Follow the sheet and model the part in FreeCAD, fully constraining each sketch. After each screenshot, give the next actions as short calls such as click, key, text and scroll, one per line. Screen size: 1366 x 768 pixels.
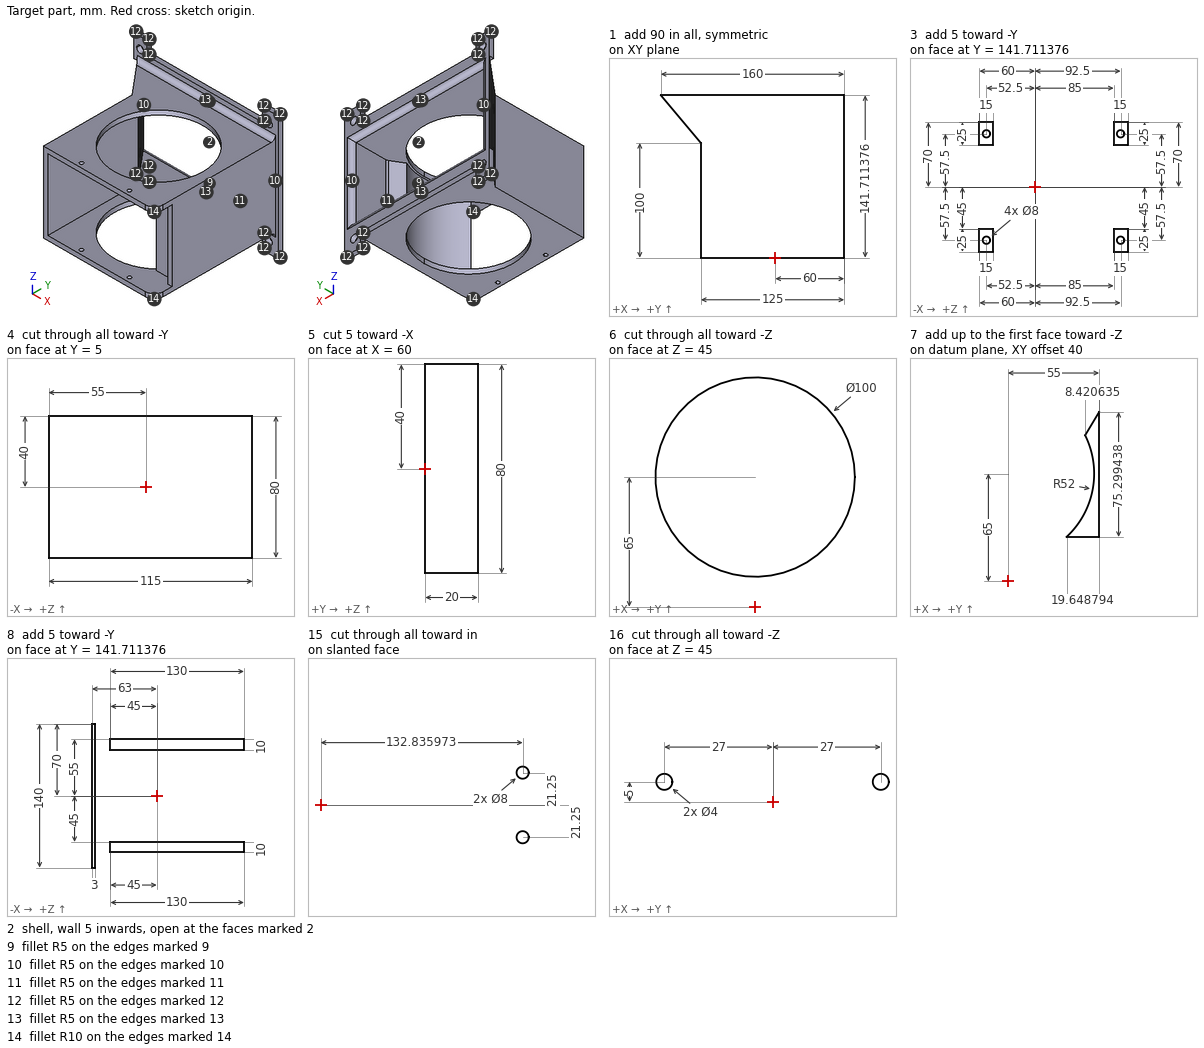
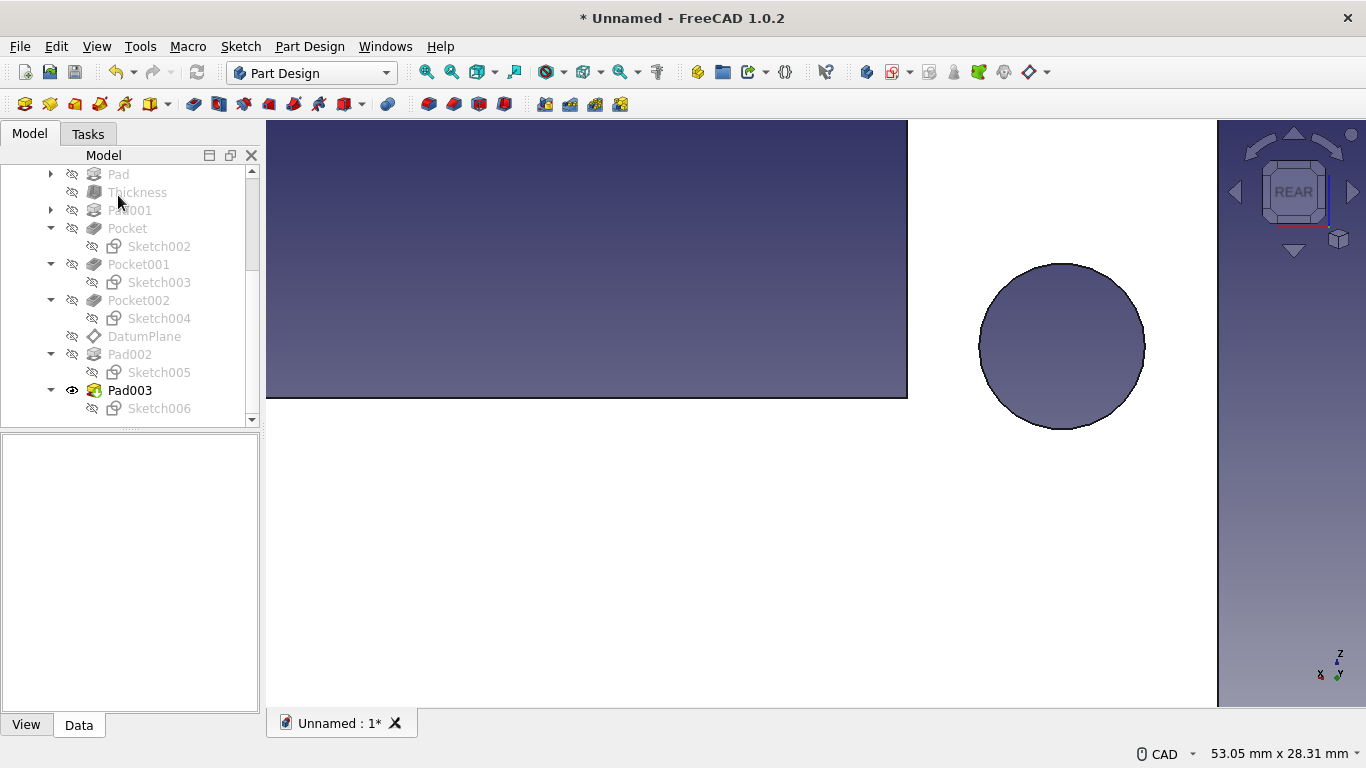
click(427, 72)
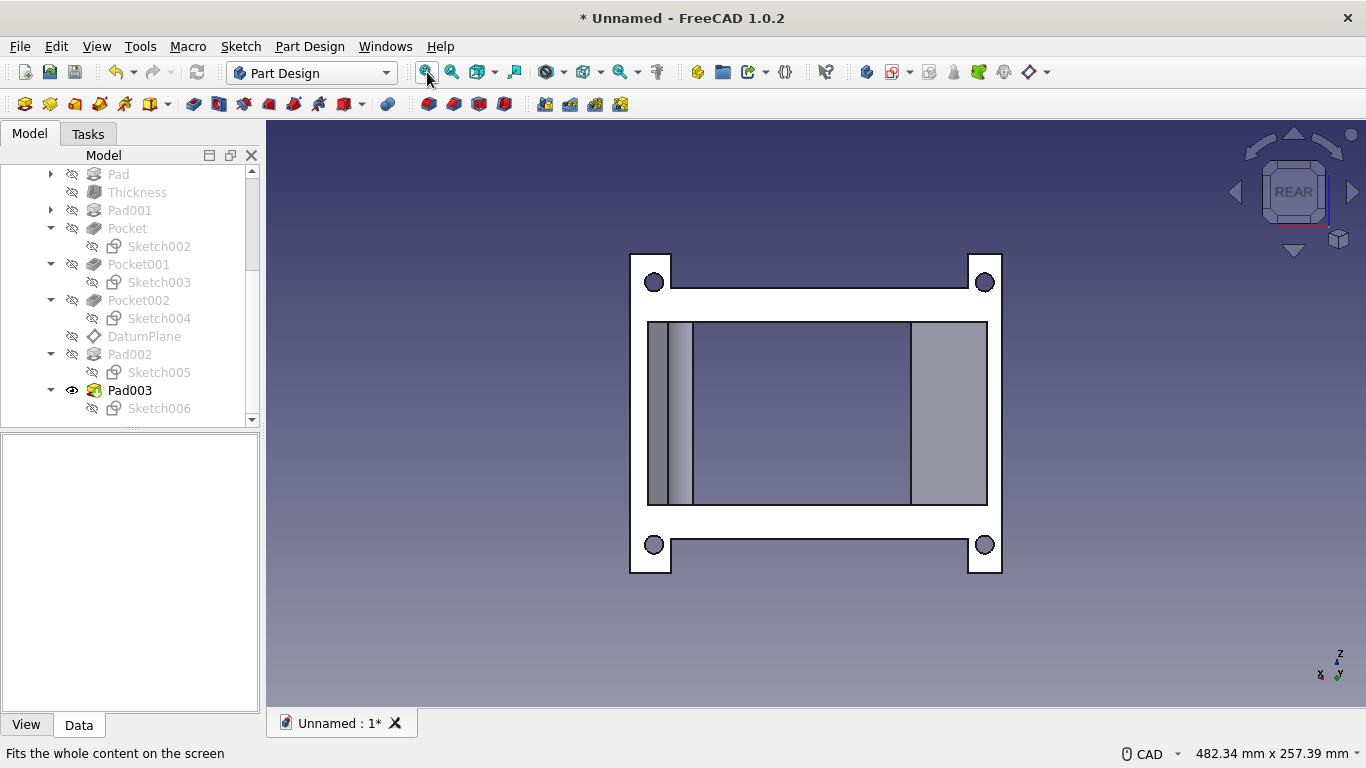
click(818, 504)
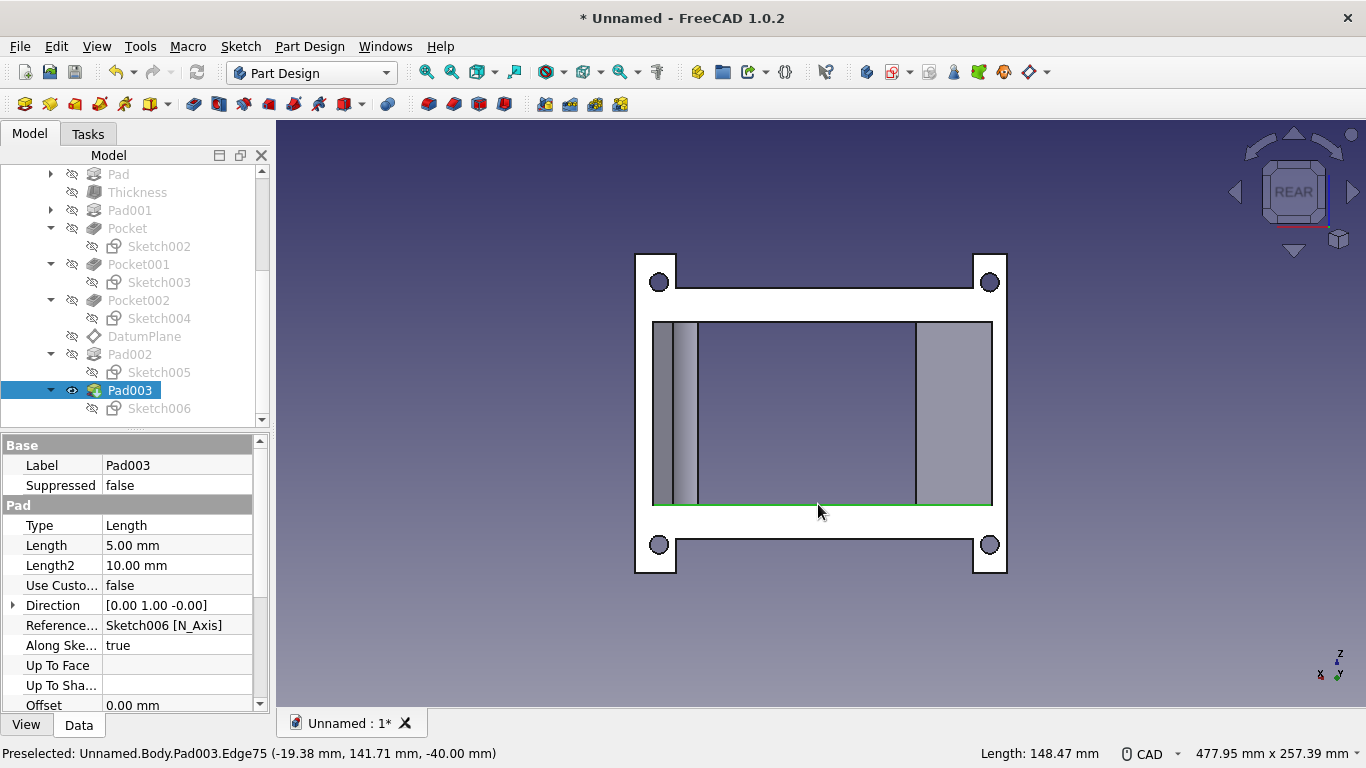
click(823, 321, ctrl)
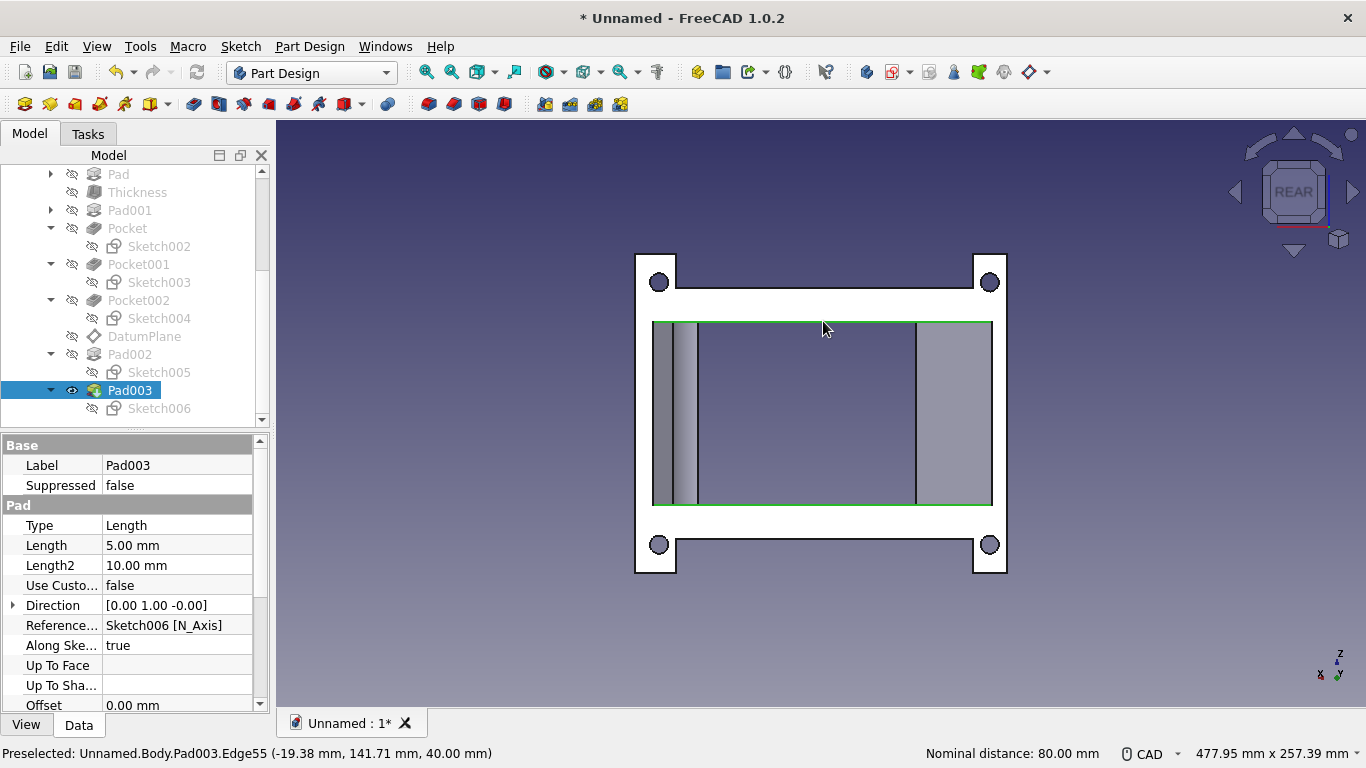
click(429, 104)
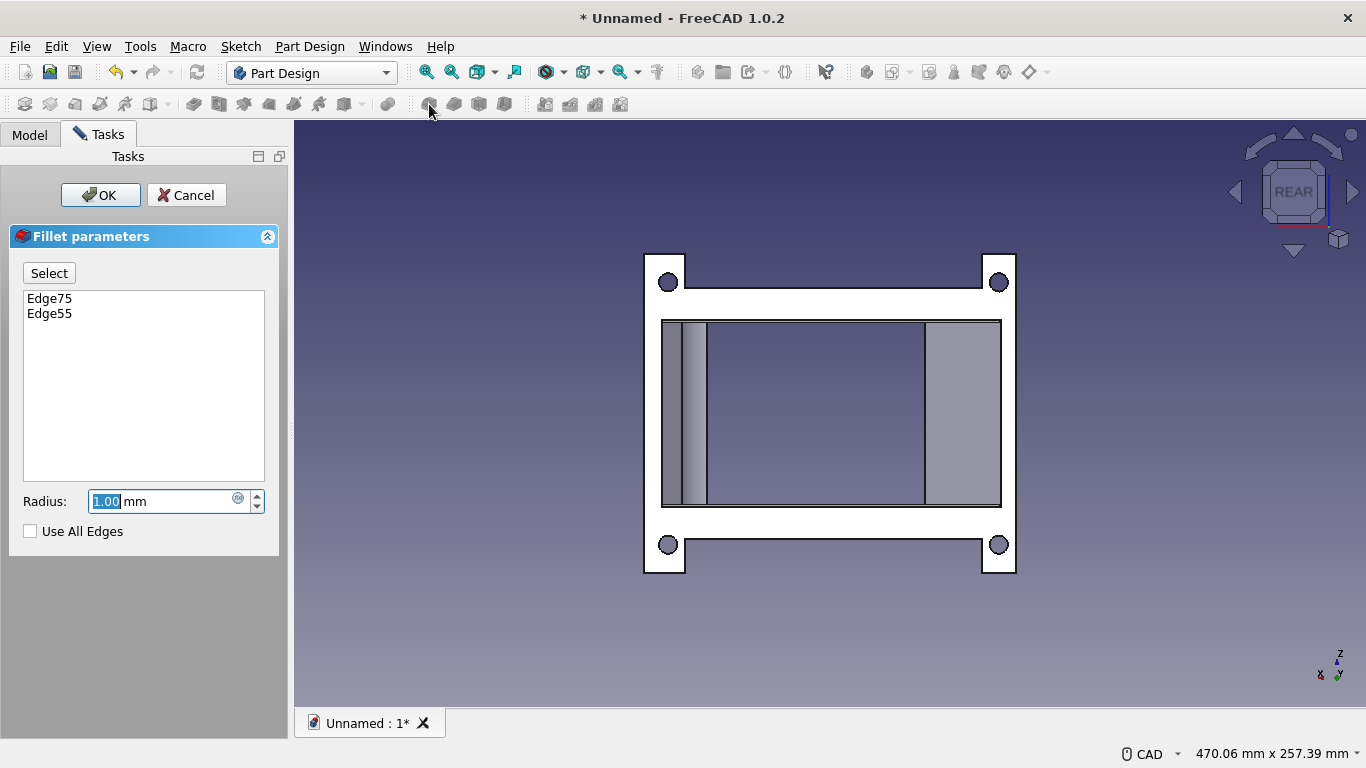
text(5)
key(Tab)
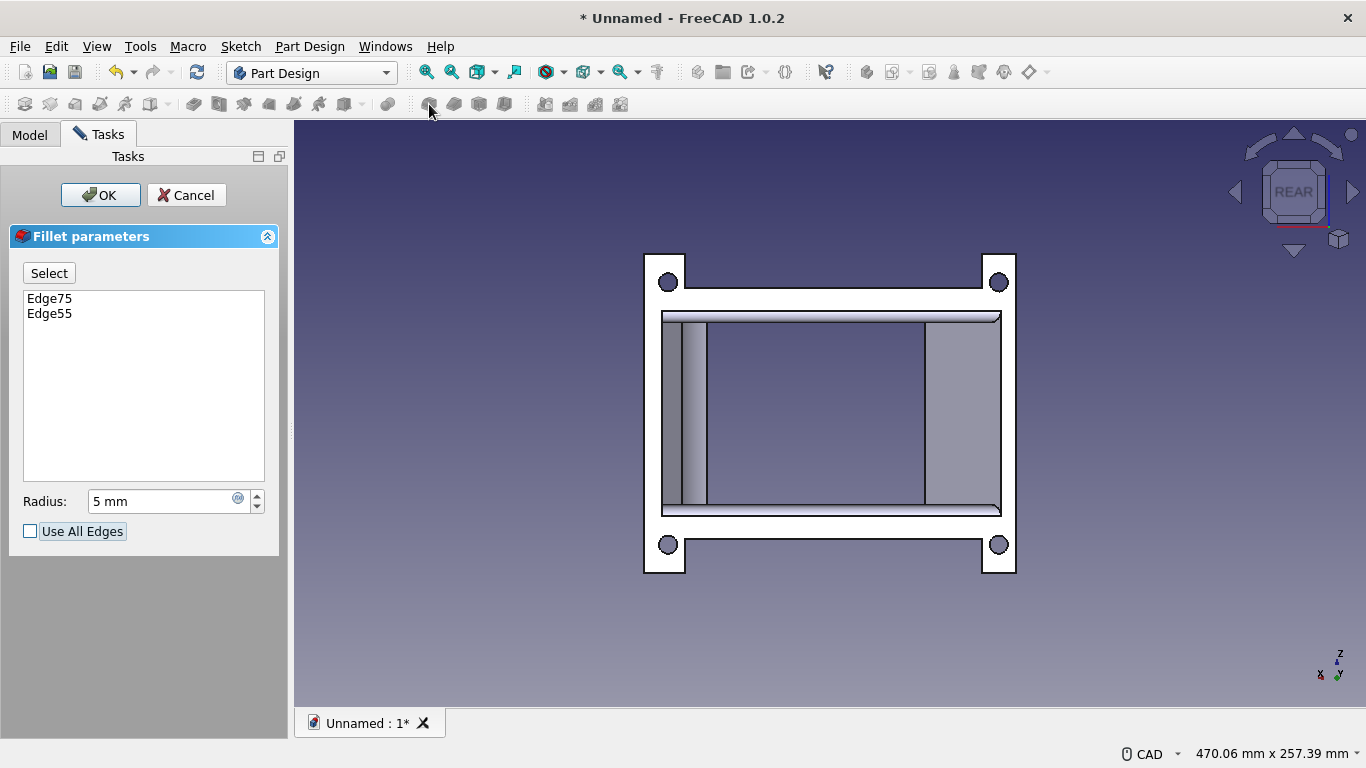
click(101, 195)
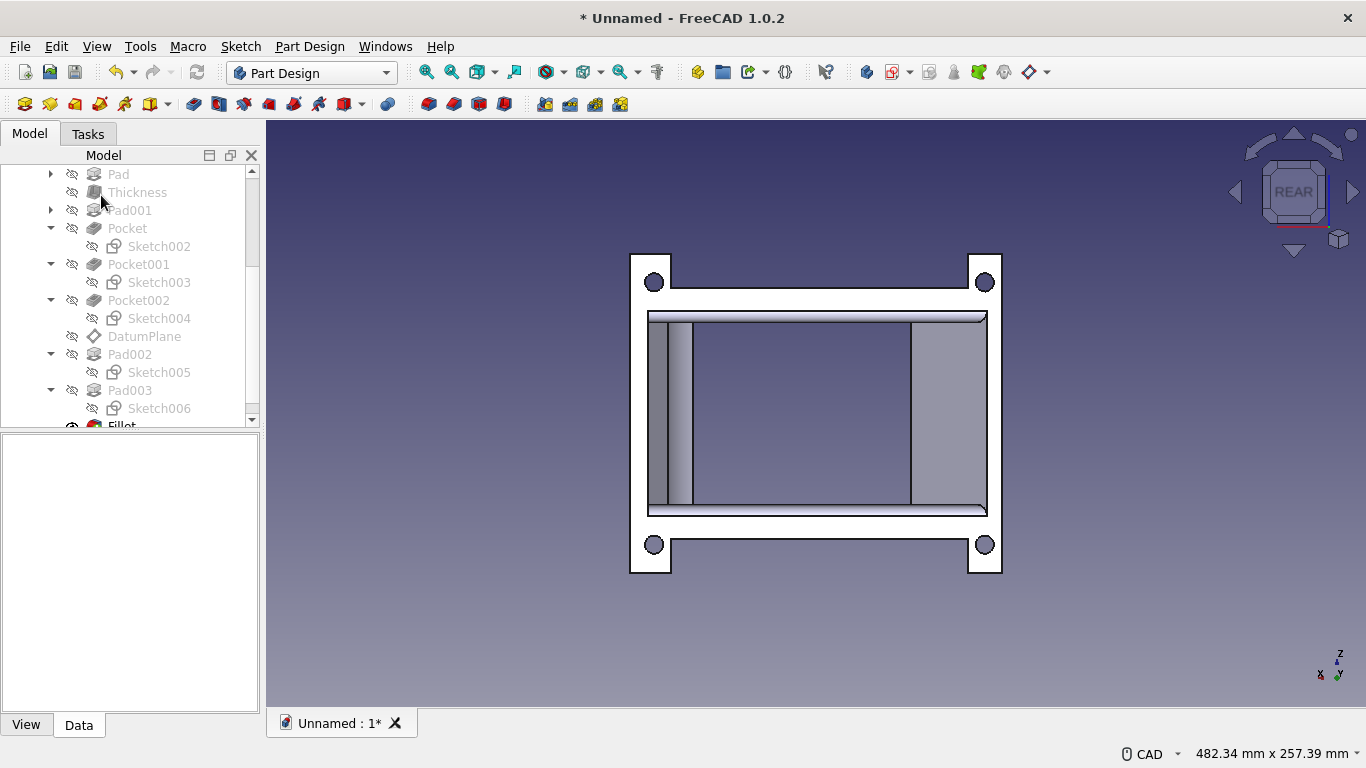
click(648, 412)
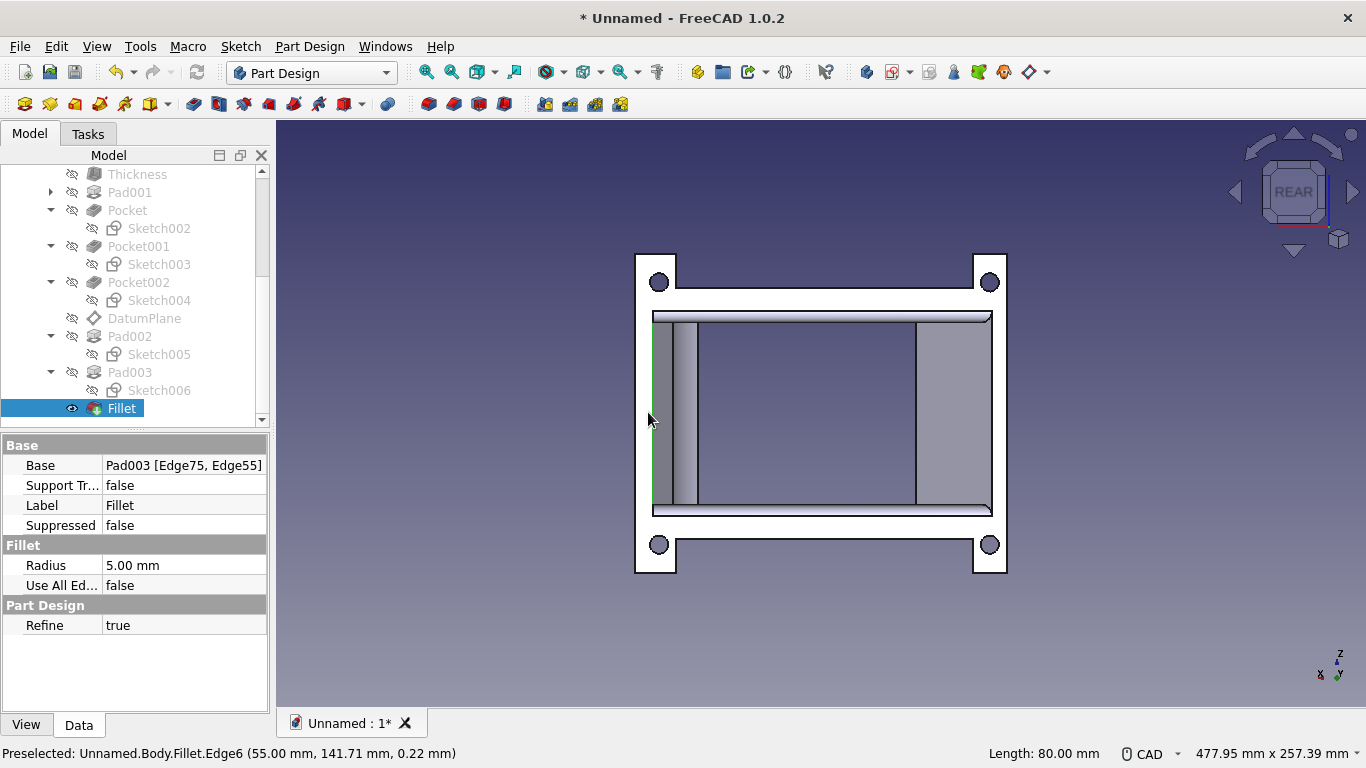
key(0)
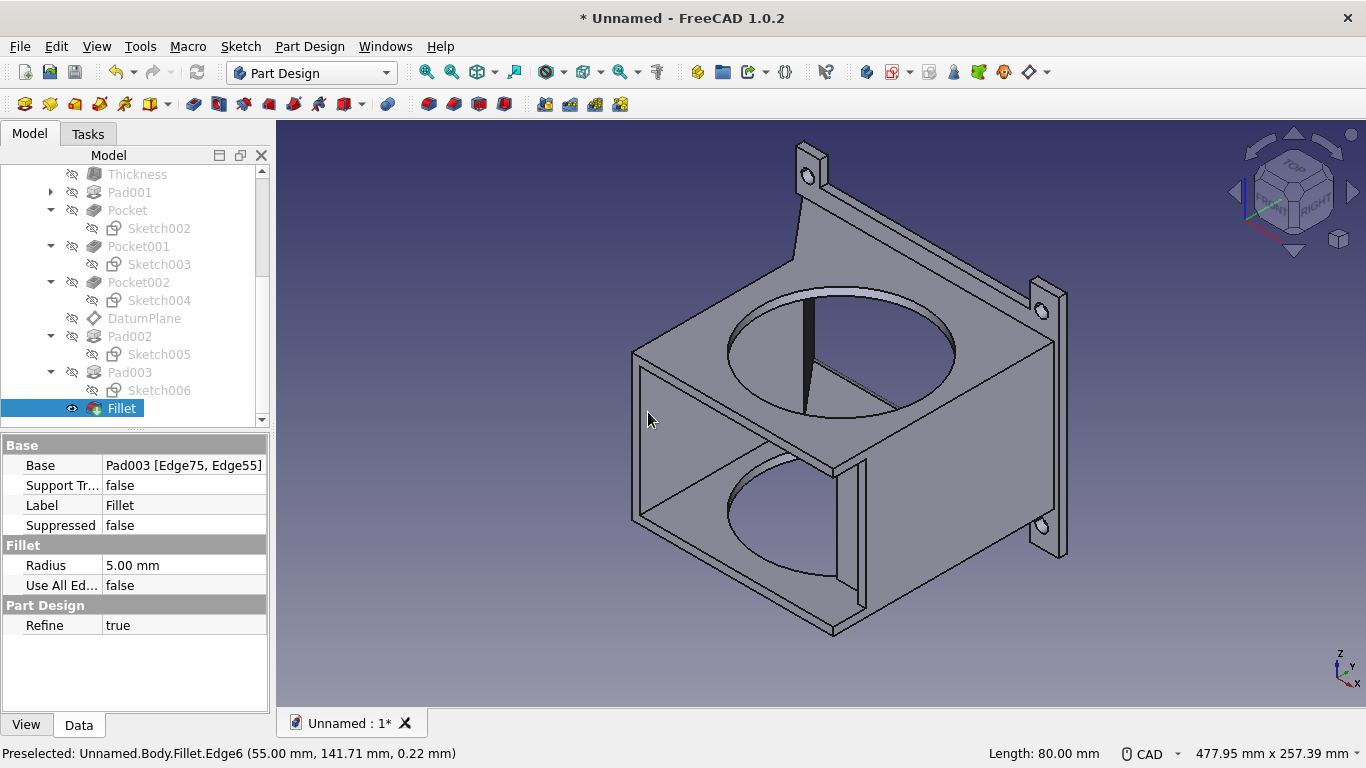
key(2)